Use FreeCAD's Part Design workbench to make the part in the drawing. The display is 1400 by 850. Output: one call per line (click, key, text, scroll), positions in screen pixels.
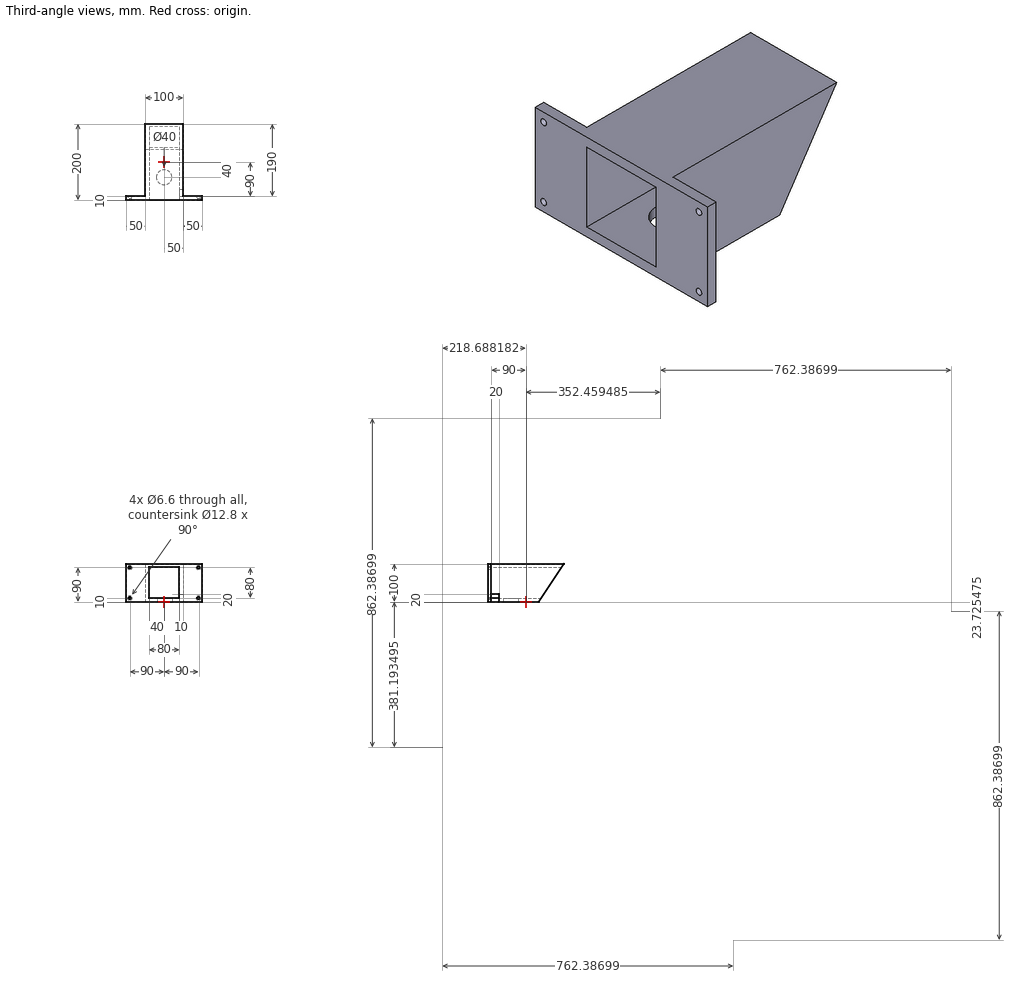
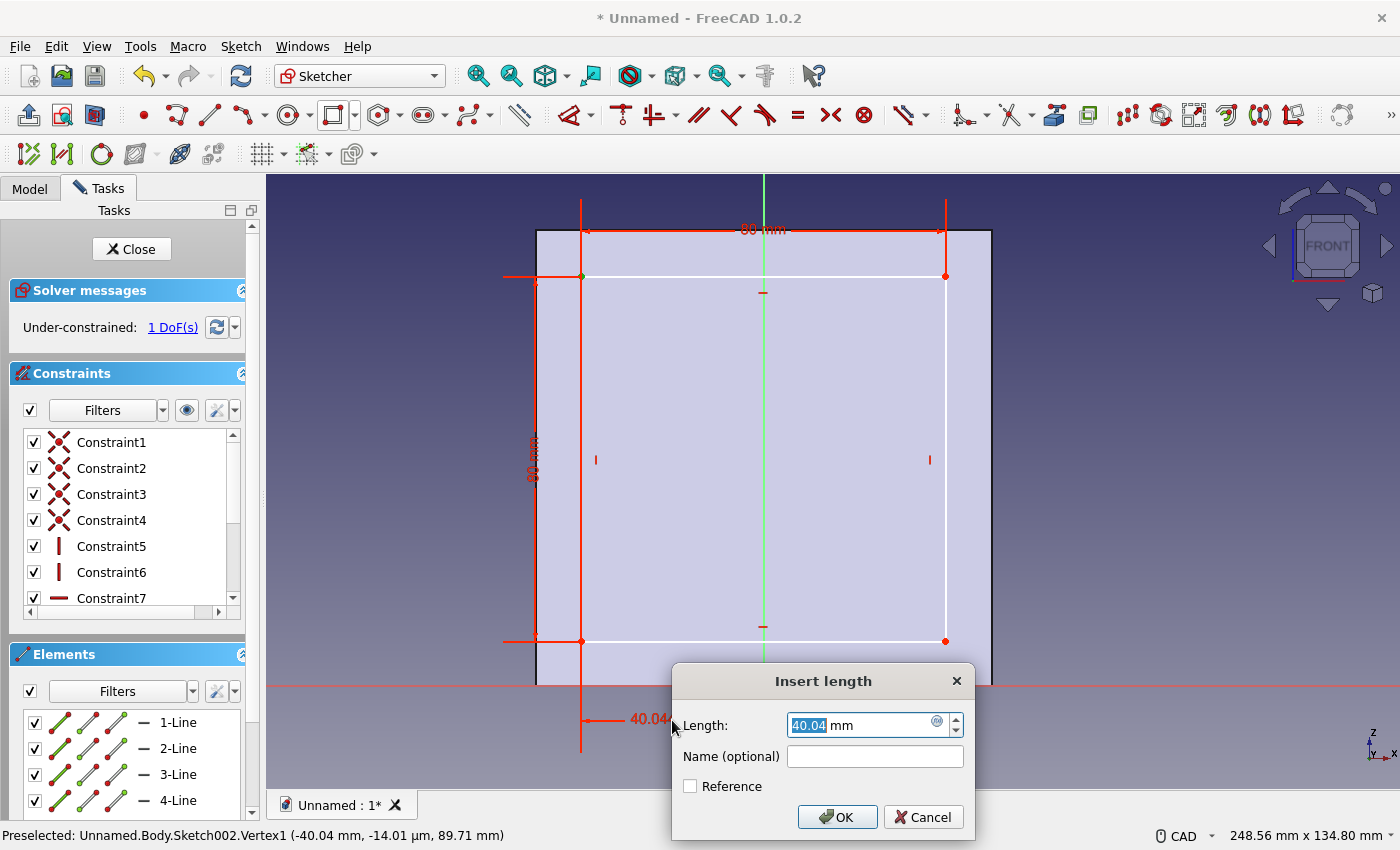
text(40)
key(Return)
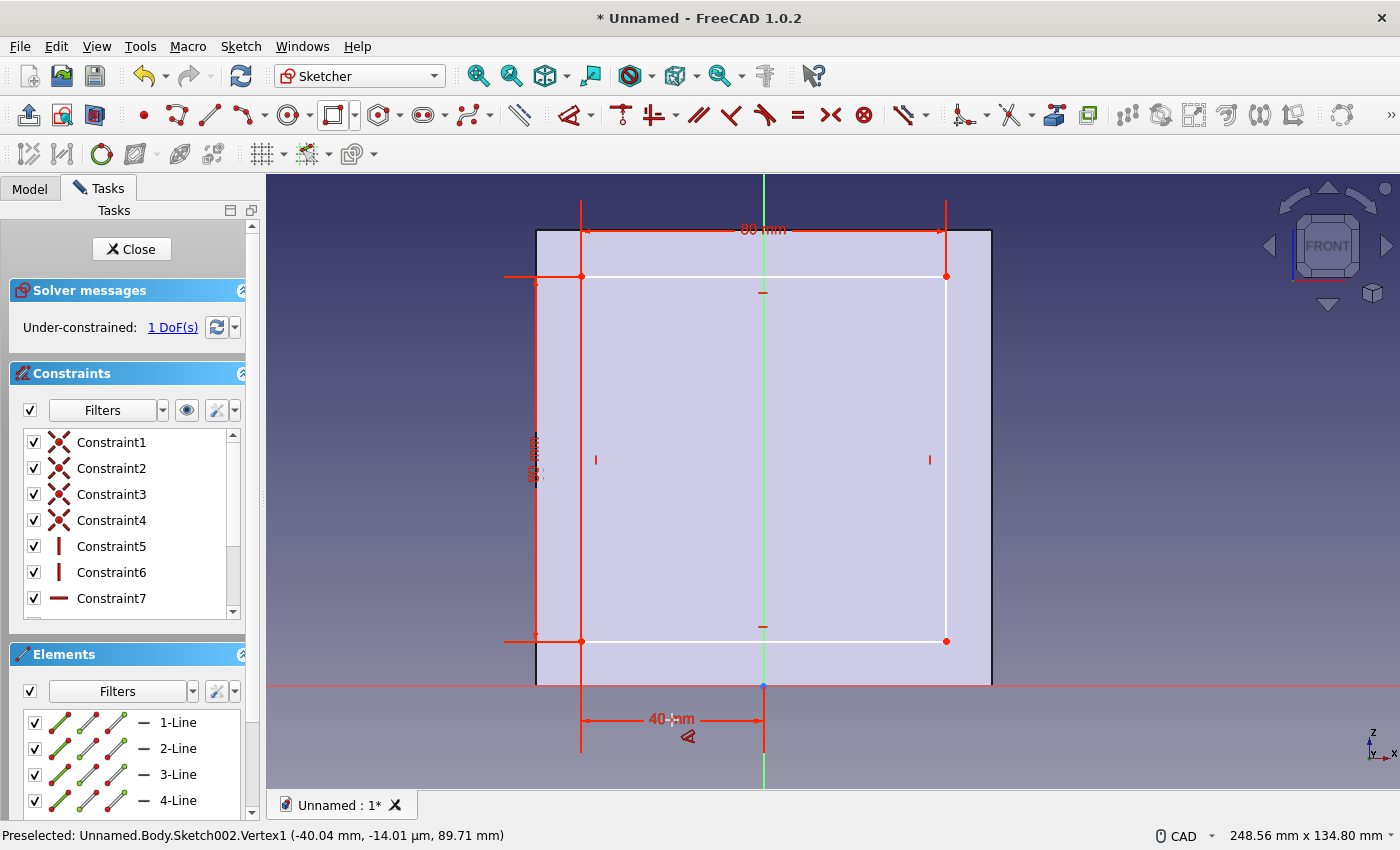
click(581, 277)
click(547, 482)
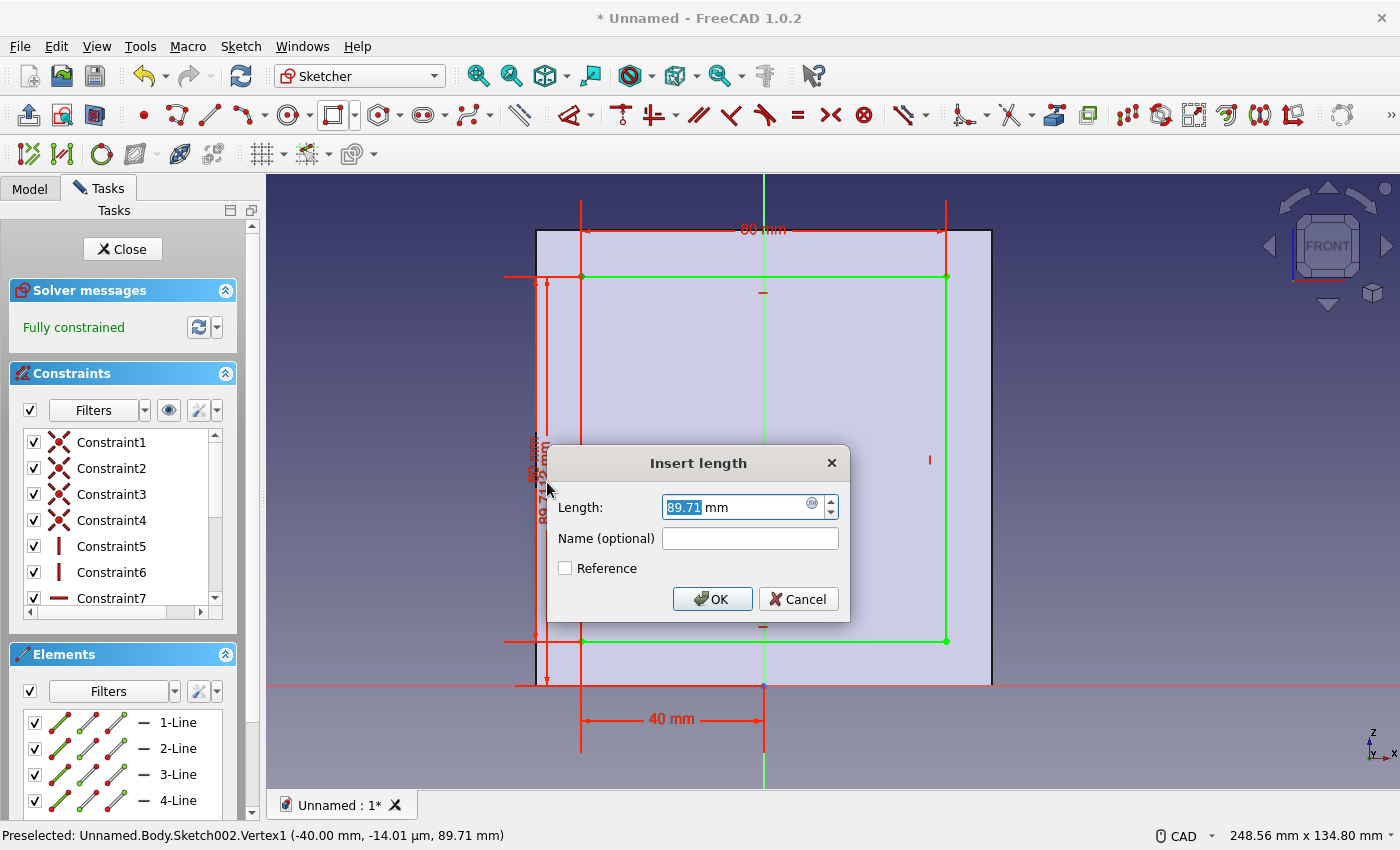
text(90)
key(Return)
key(Escape)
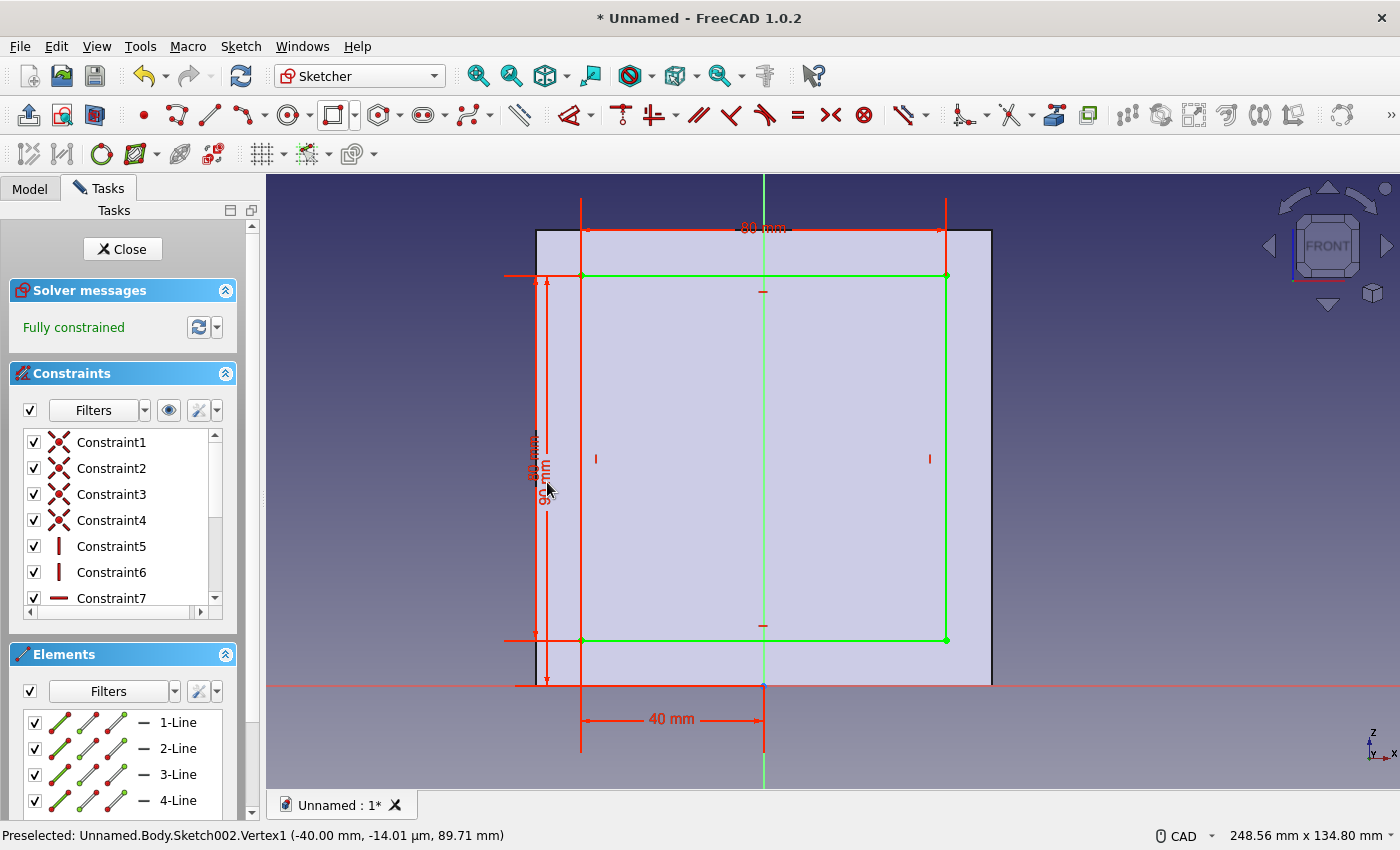
click(123, 249)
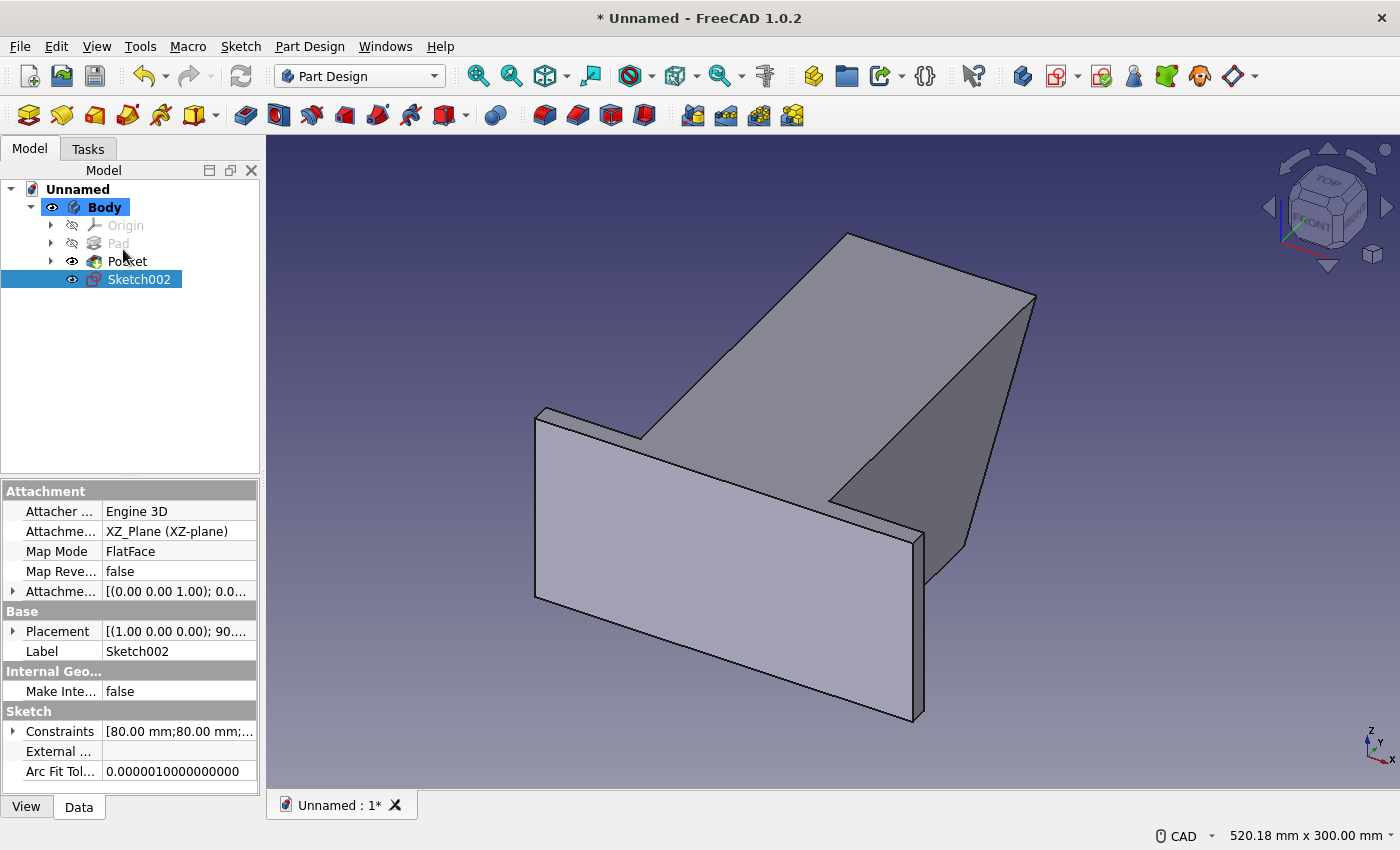
click(246, 116)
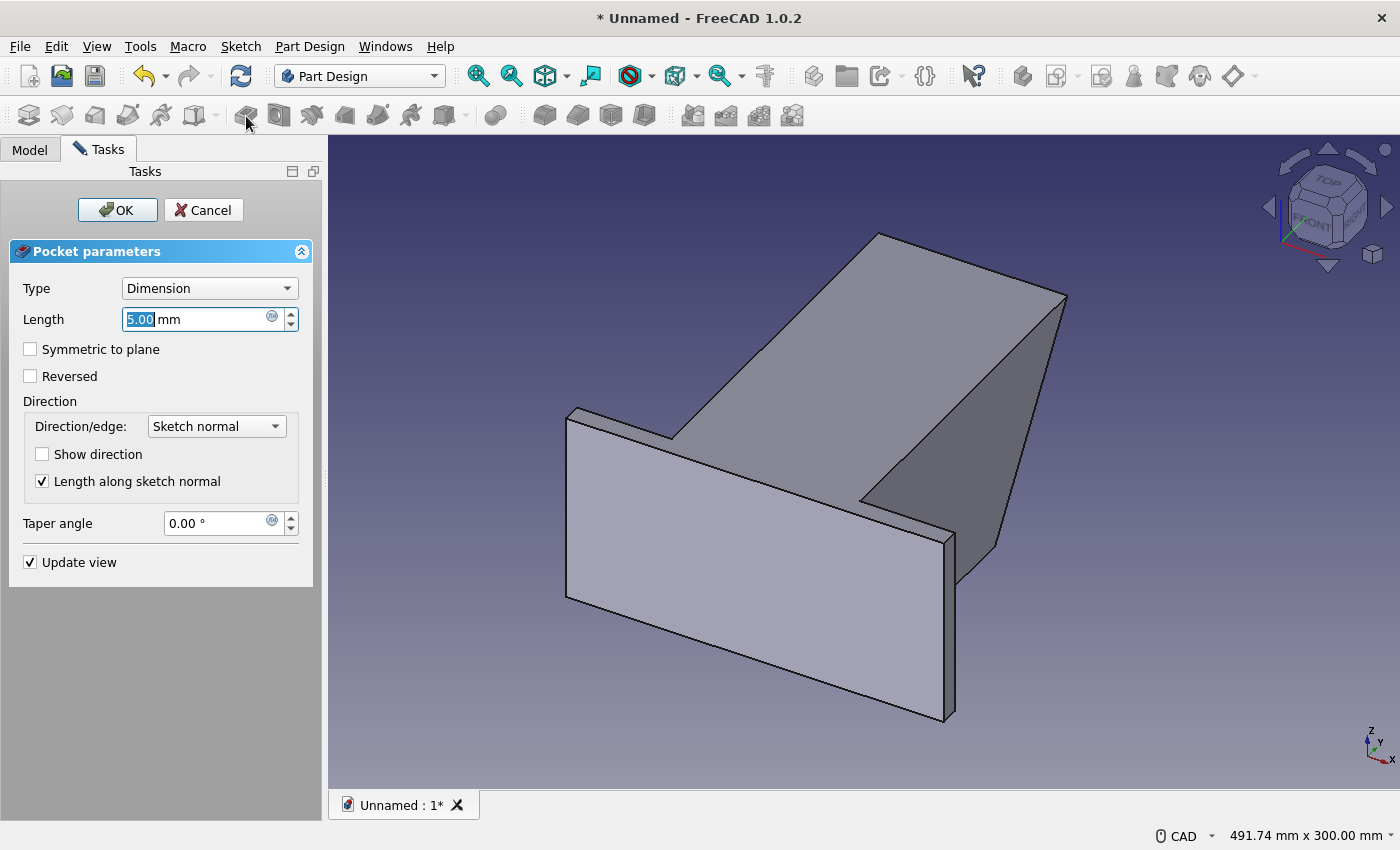
text(200)
key(Tab)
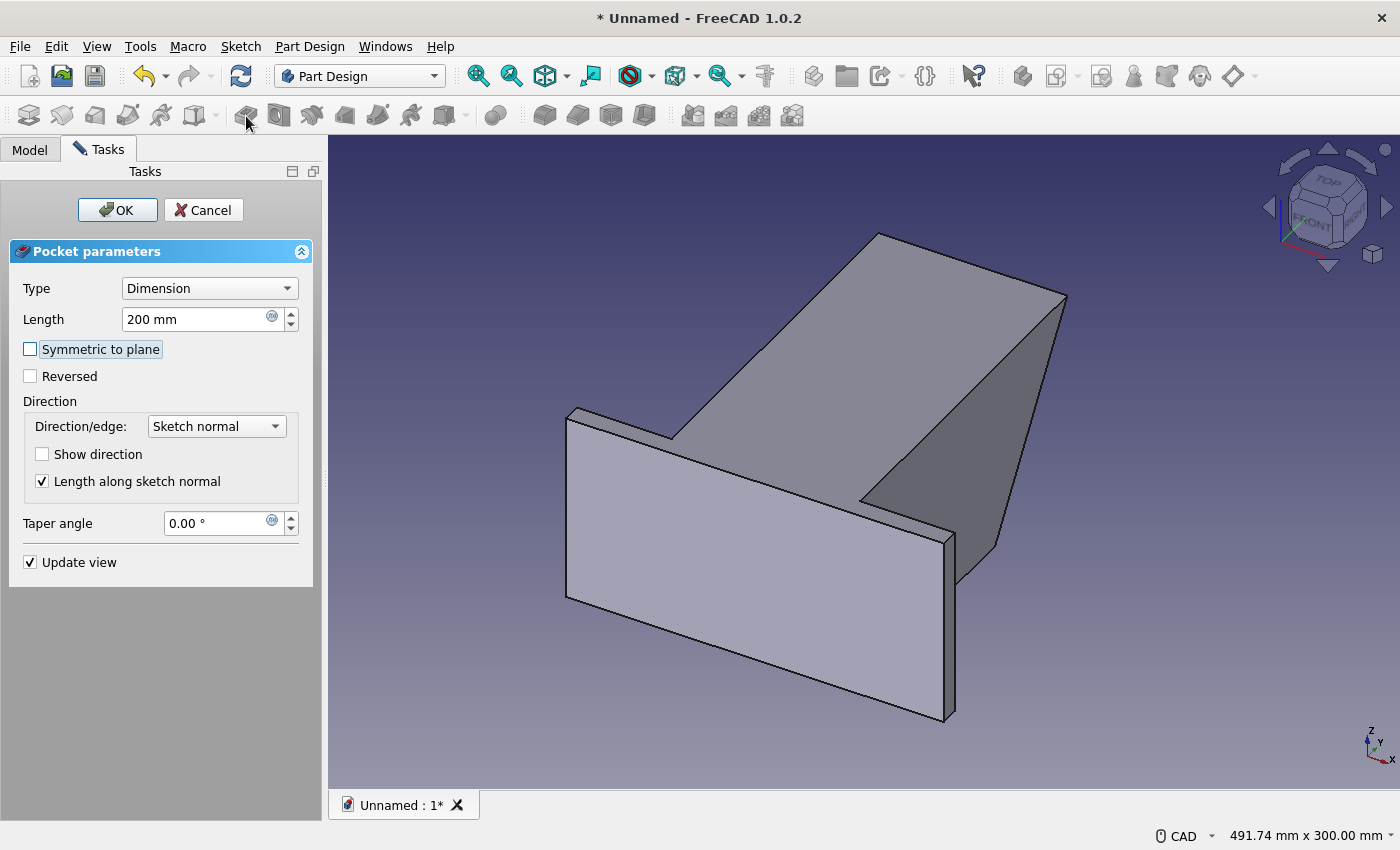
click(31, 349)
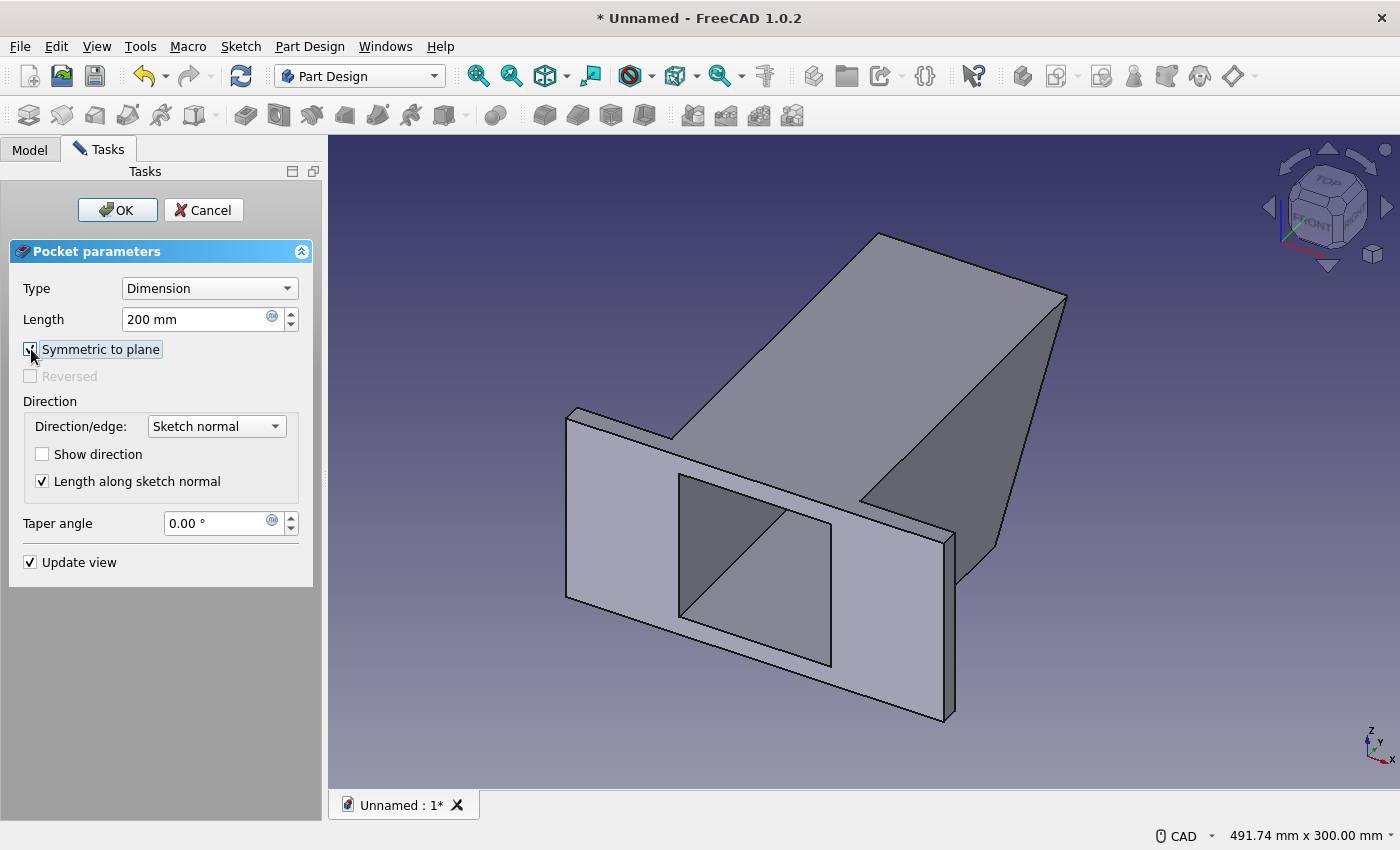
click(118, 210)